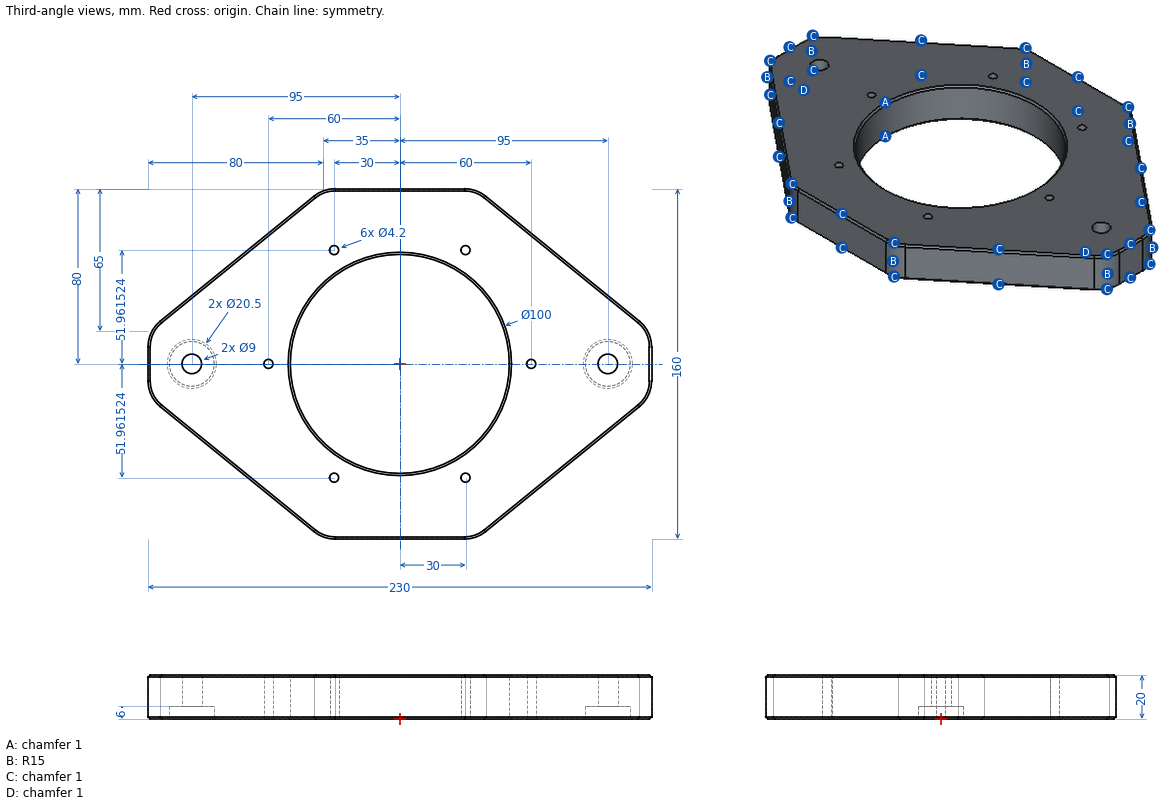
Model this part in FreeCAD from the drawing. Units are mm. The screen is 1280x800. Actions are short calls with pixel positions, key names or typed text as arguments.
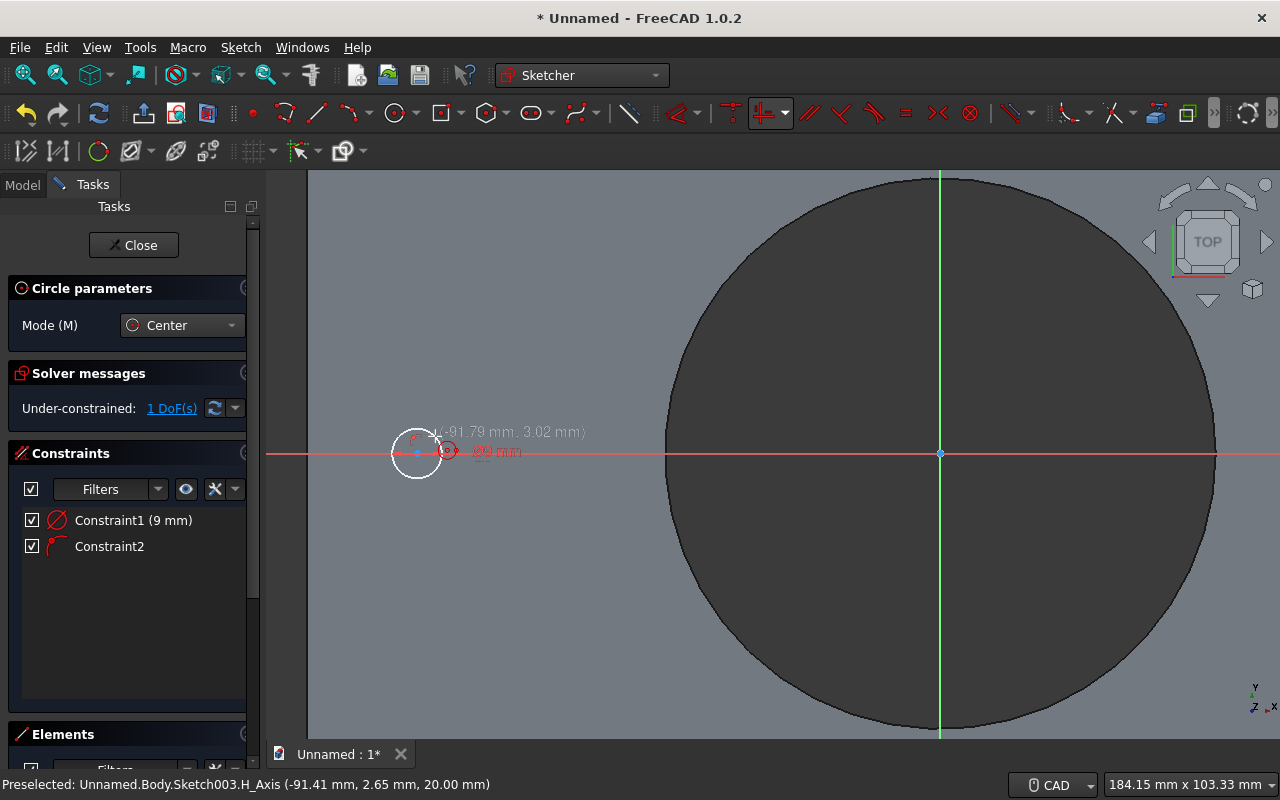
scroll(418, 456, down, 3)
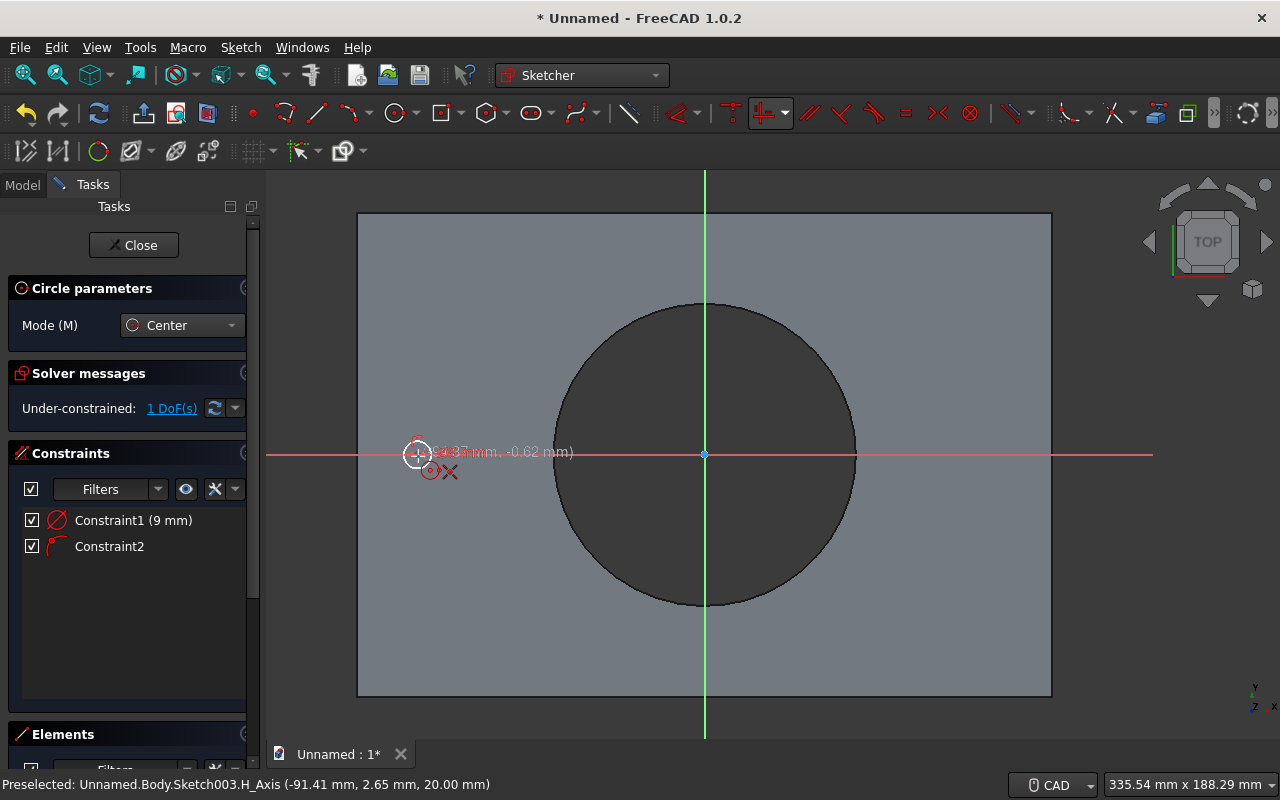
scroll(992, 455, up, 3)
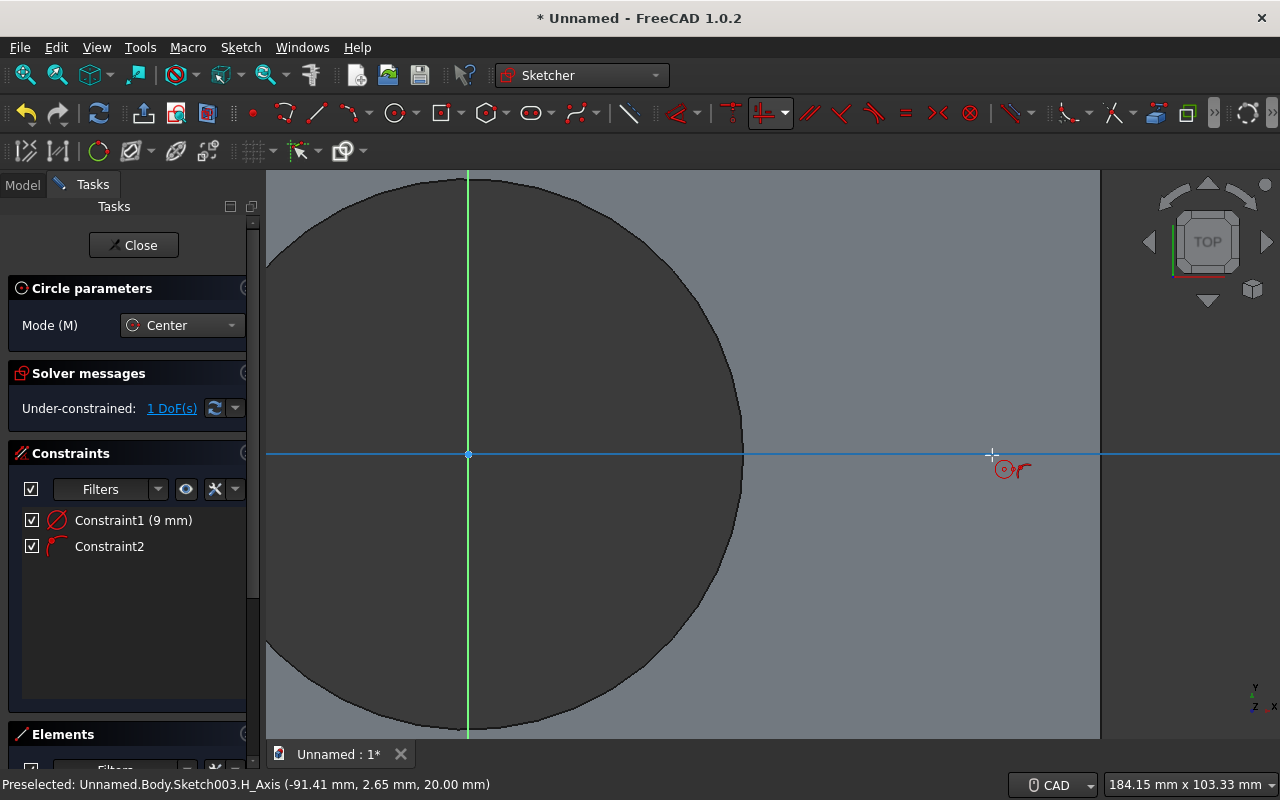
click(991, 454)
move(1009, 437)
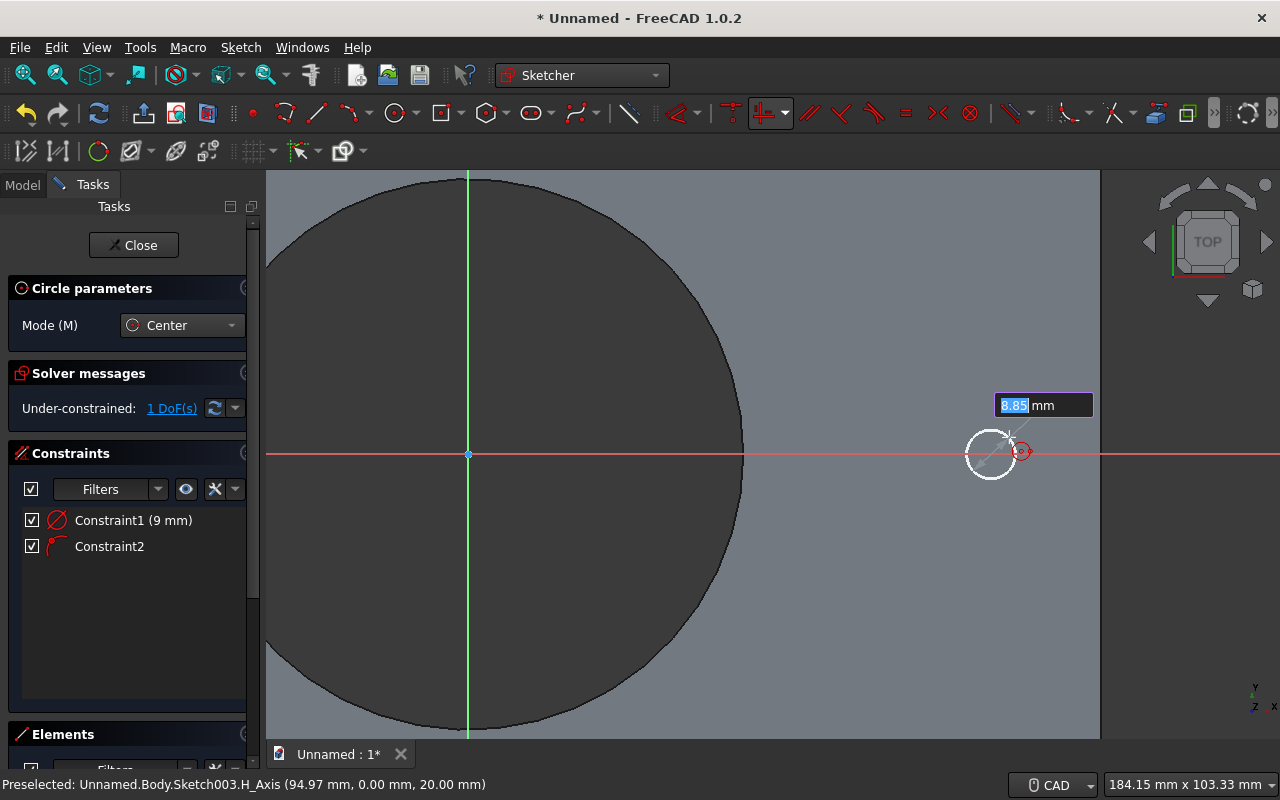
text(9)
key(Return)
key(Escape)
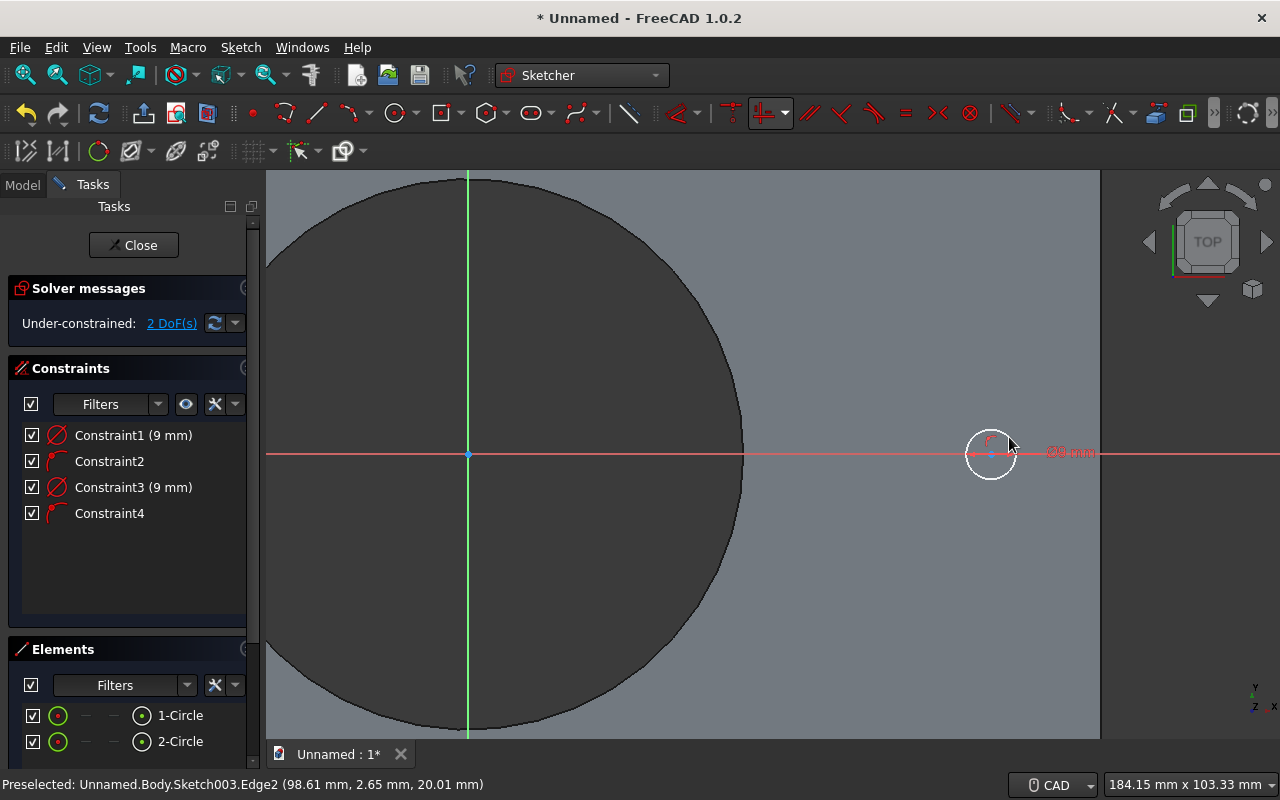
click(676, 114)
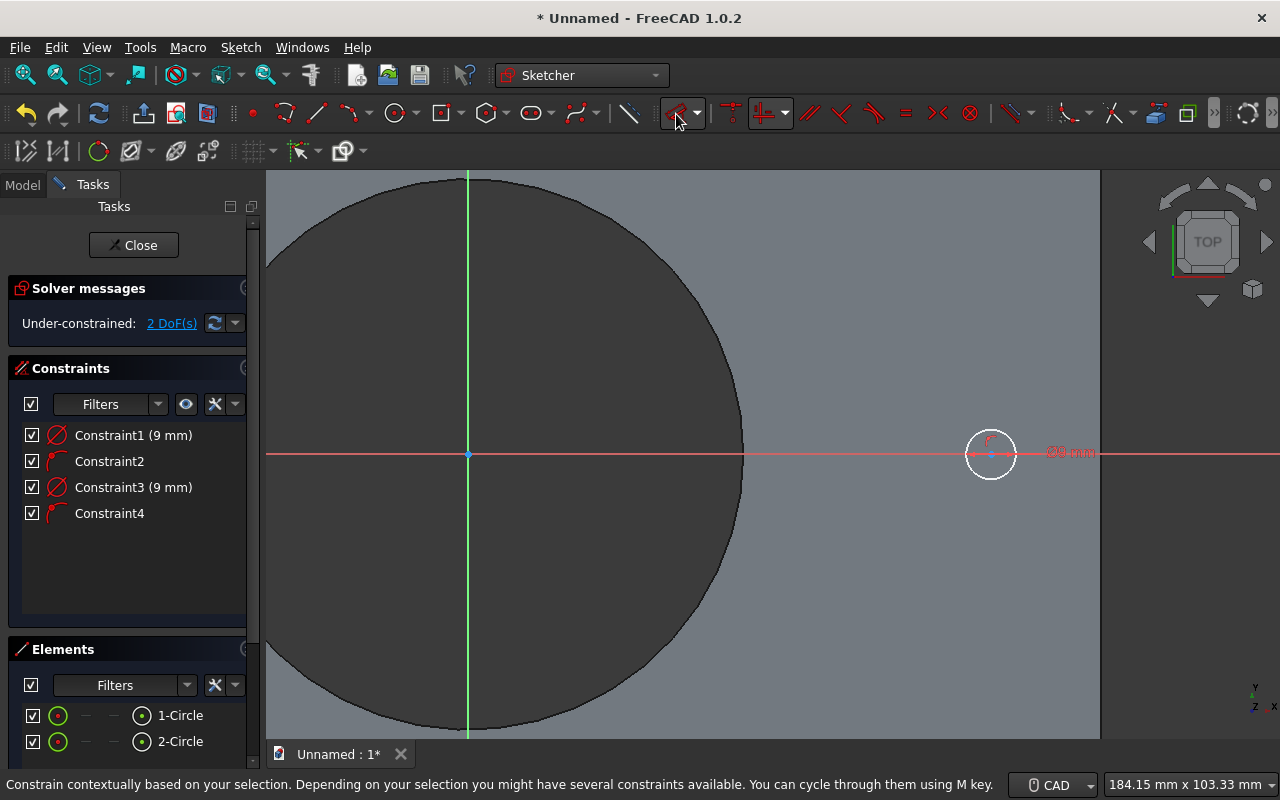
scroll(992, 455, down, 3)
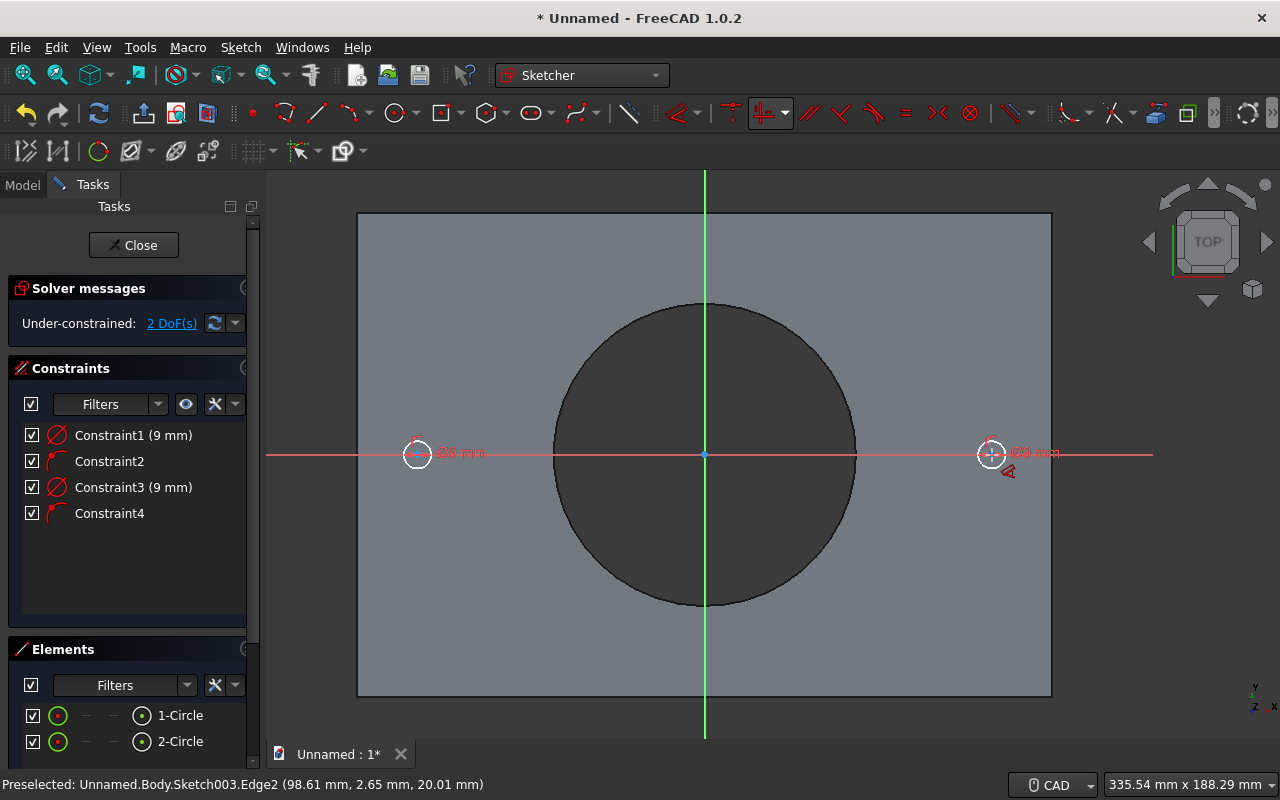
click(418, 455)
click(561, 489)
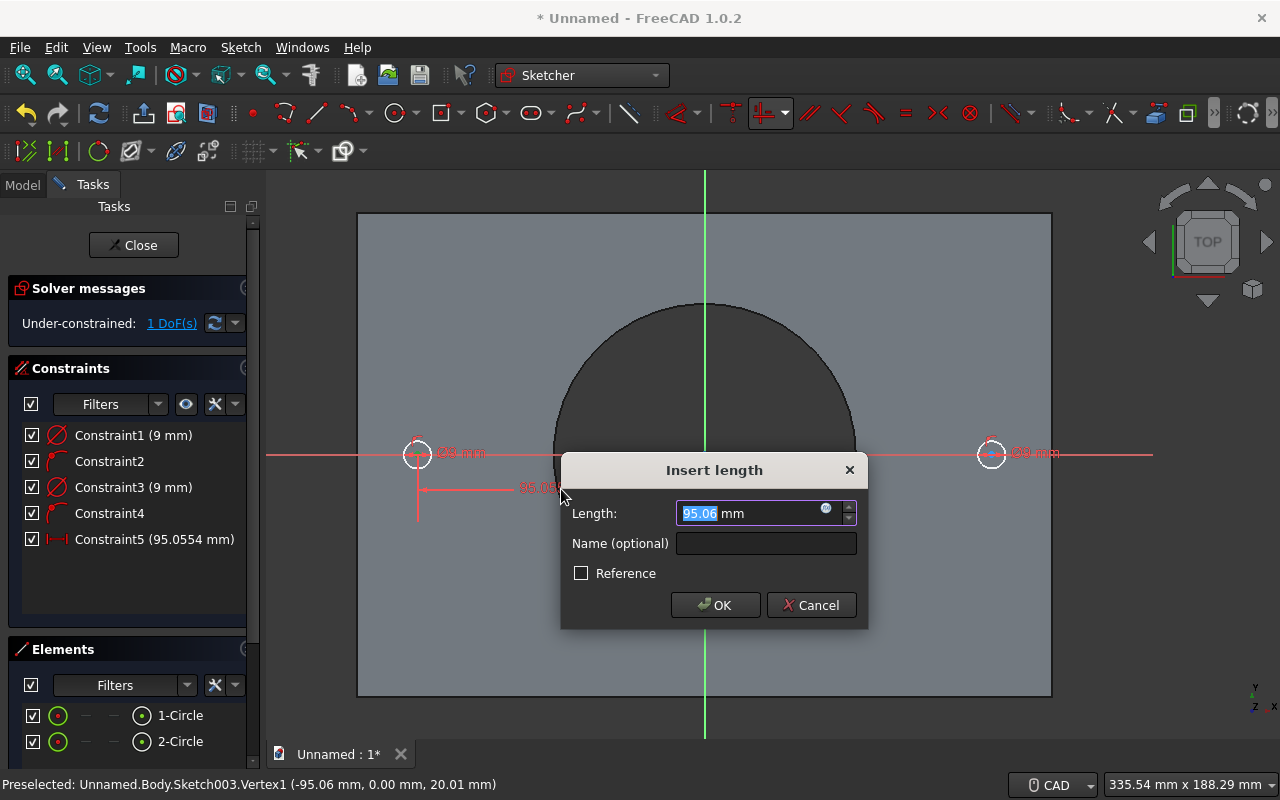
text(95)
key(Return)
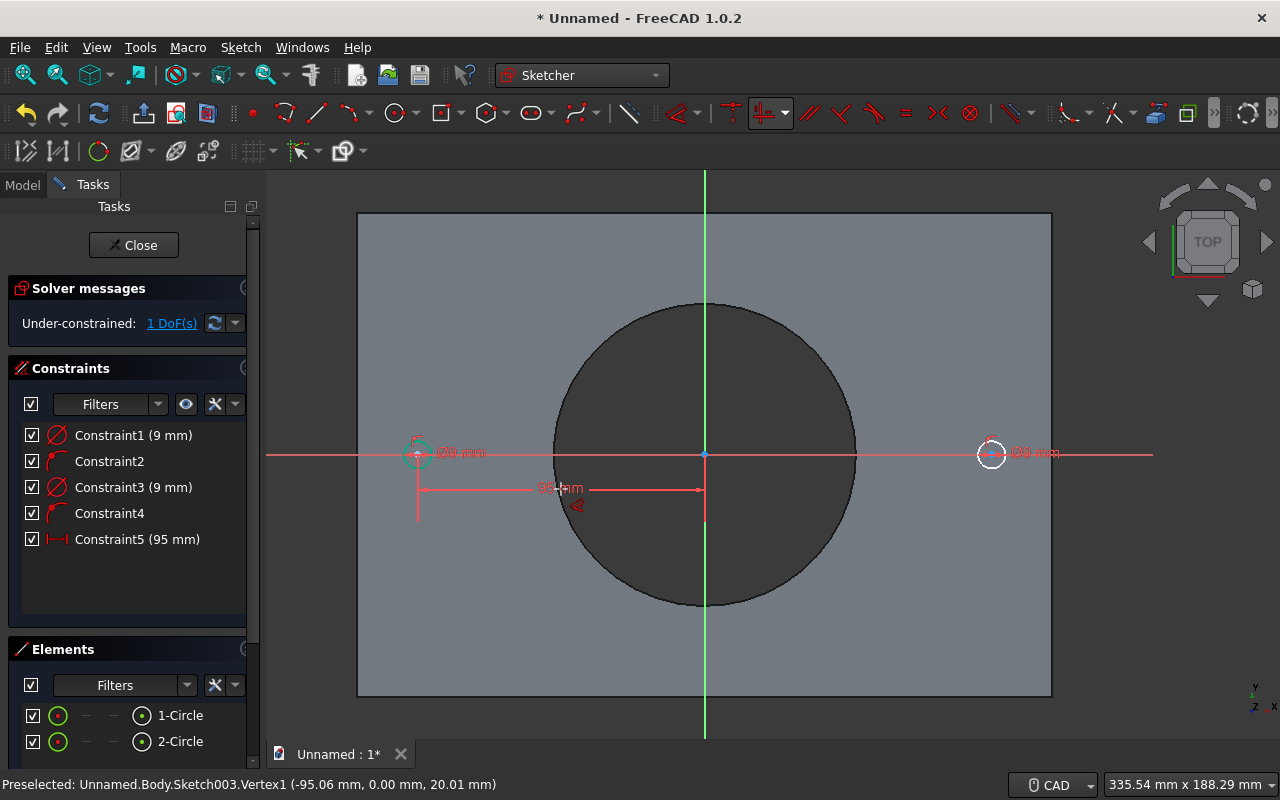
click(992, 455)
click(848, 489)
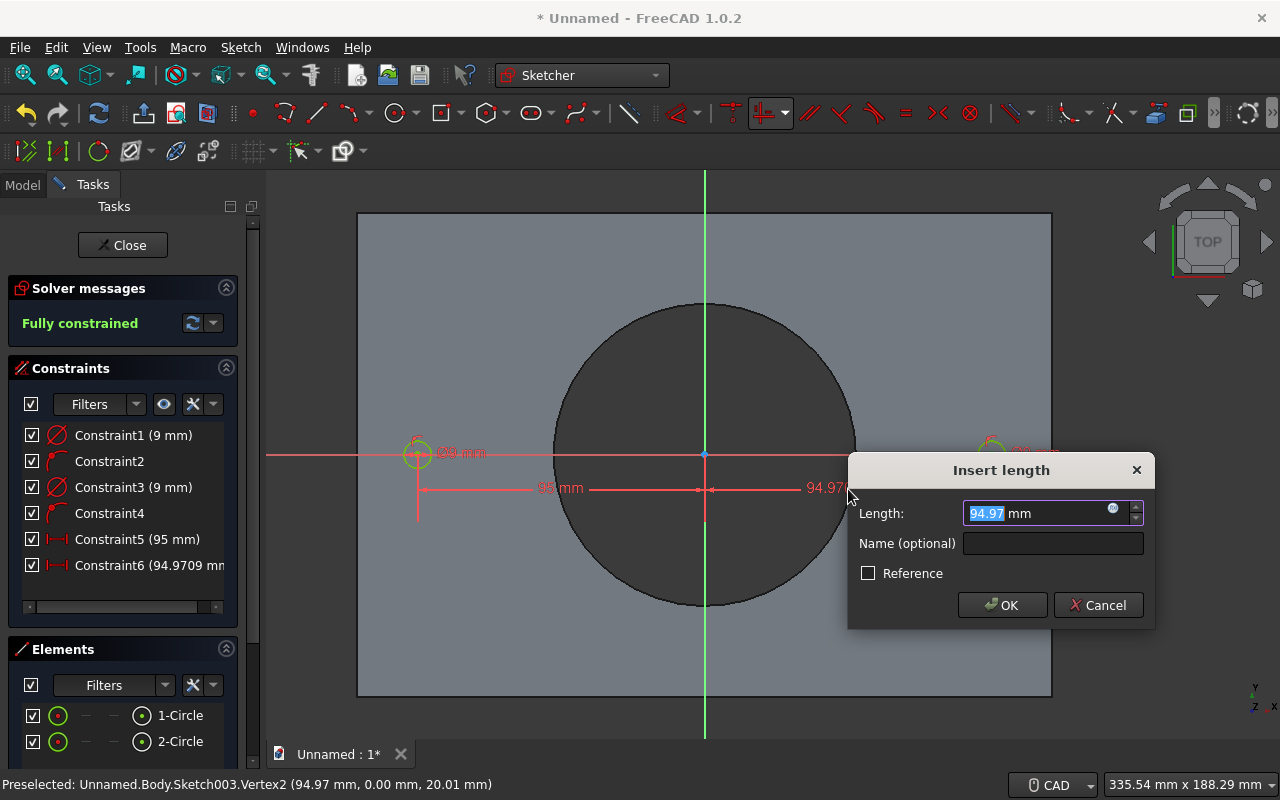
text(95)
key(Return)
key(Escape)